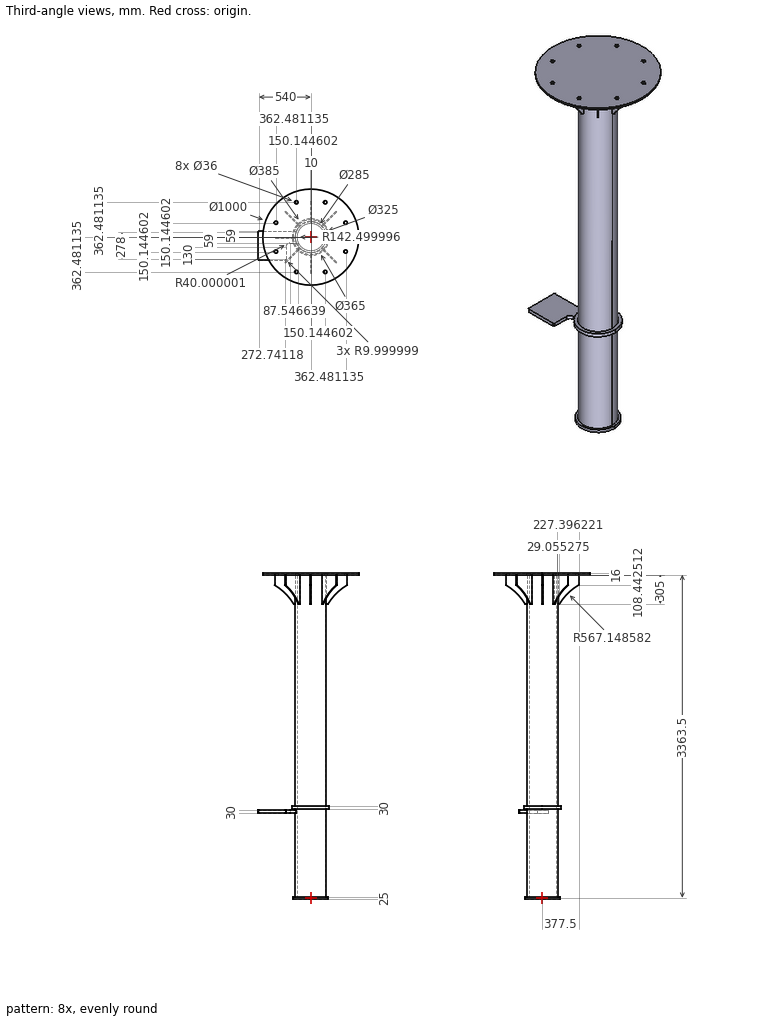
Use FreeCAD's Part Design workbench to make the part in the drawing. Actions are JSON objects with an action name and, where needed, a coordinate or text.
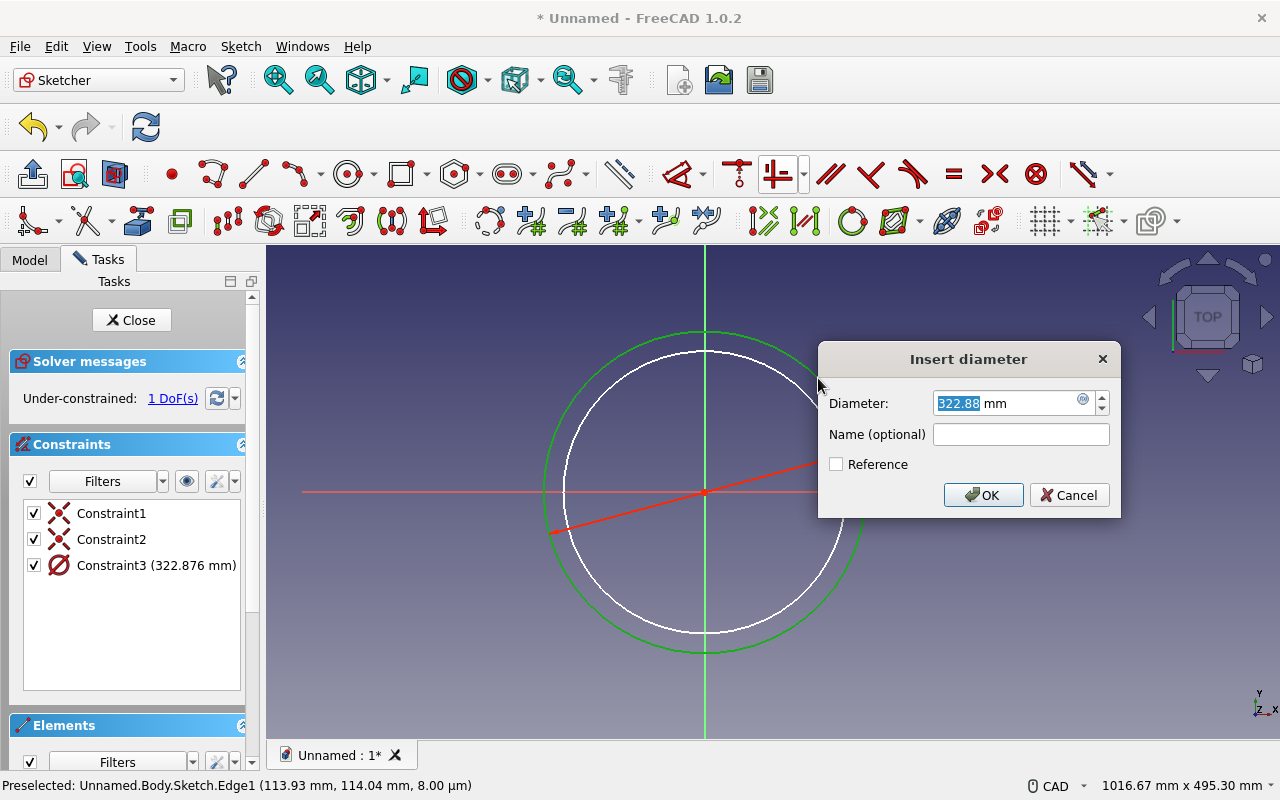
{"action": "type", "text": "325"}
{"action": "key", "text": "Return"}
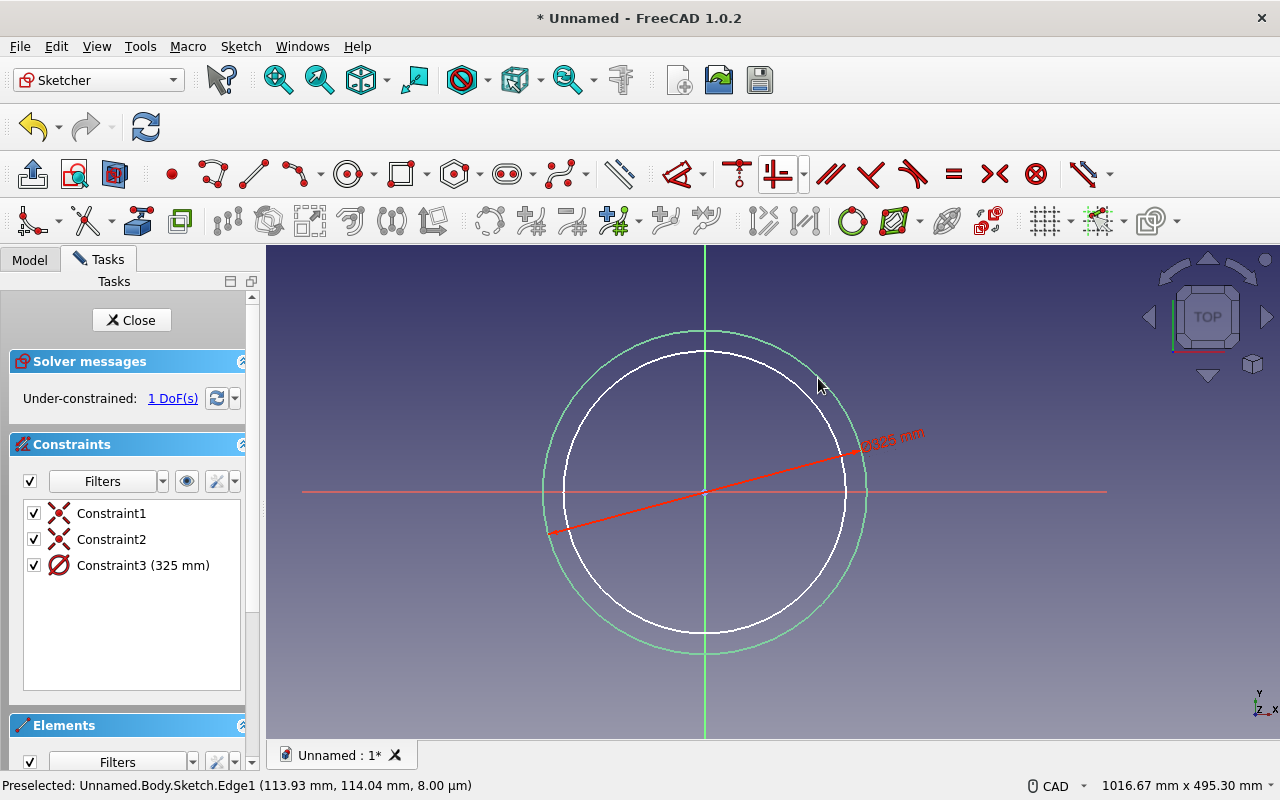
{"action": "left_click", "coordinate": [804, 392]}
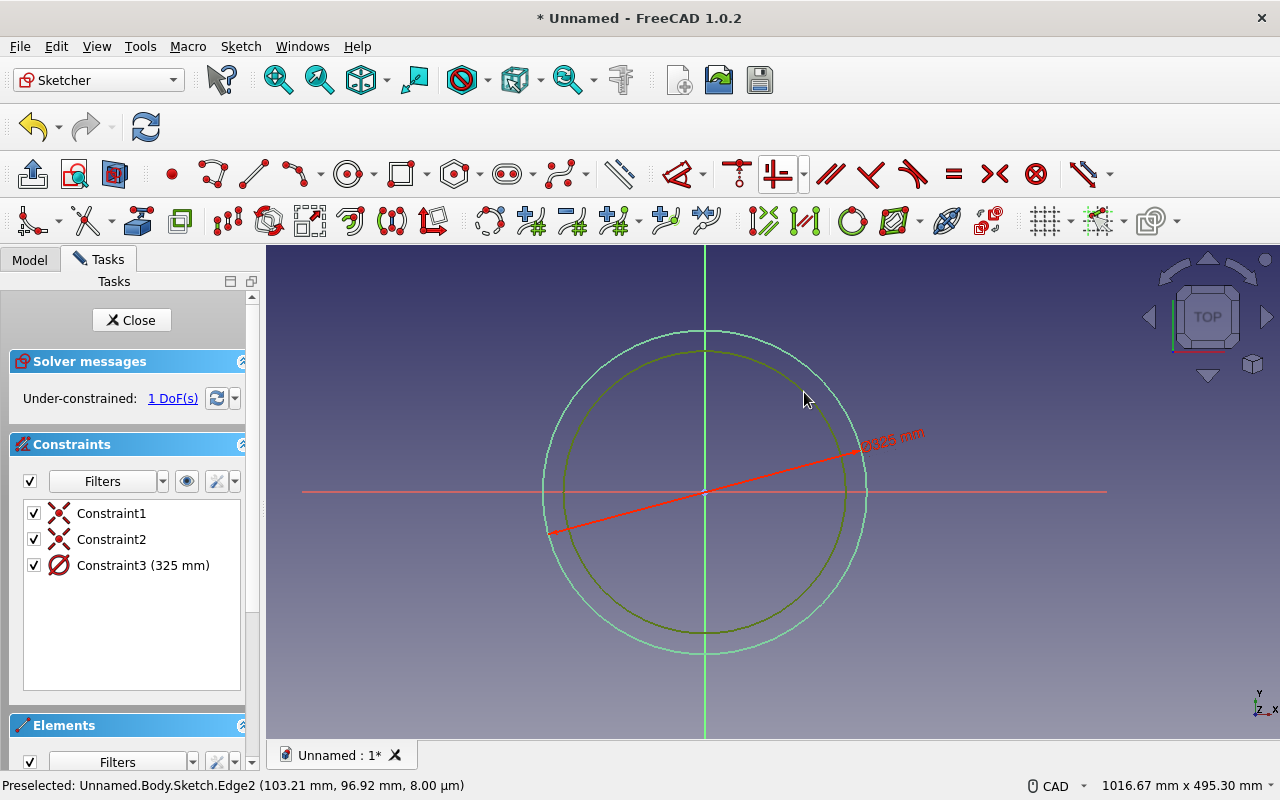
{"action": "key", "text": "k o"}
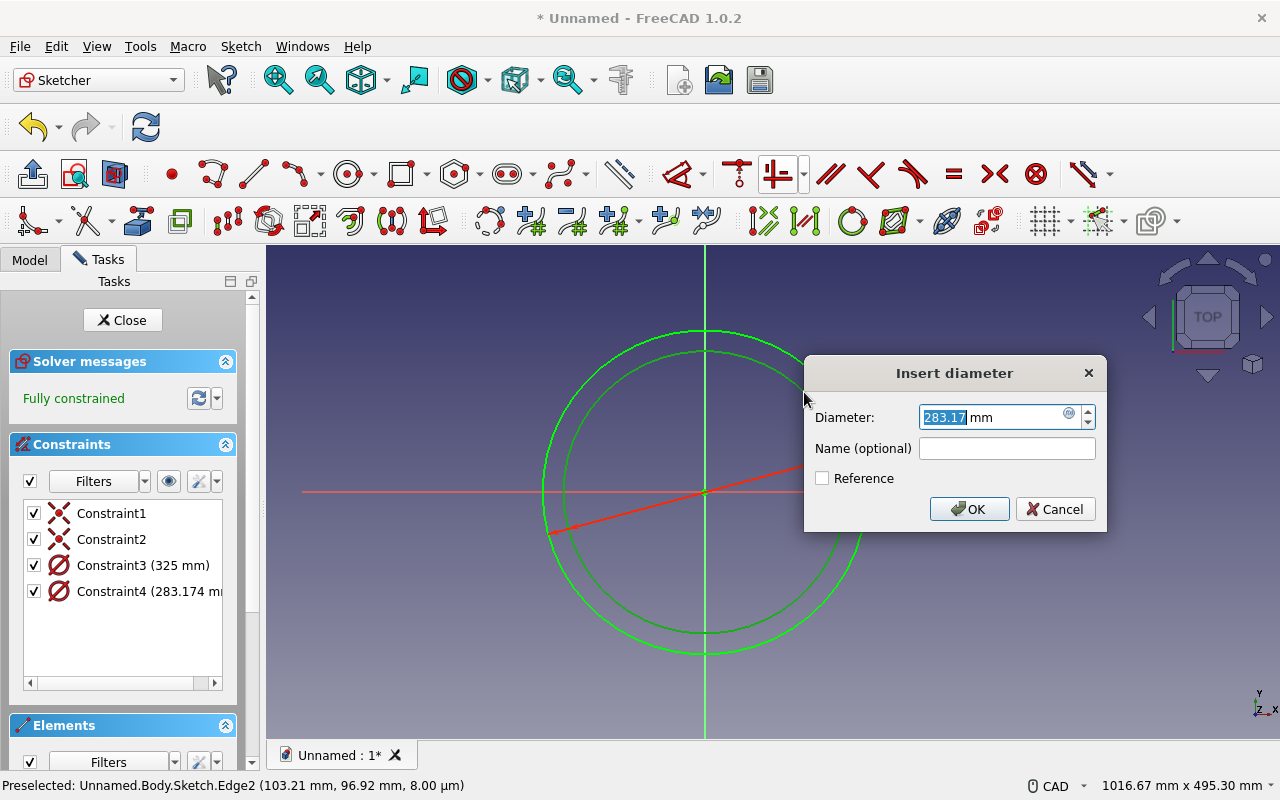
{"action": "type", "text": "285"}
{"action": "key", "text": "Return"}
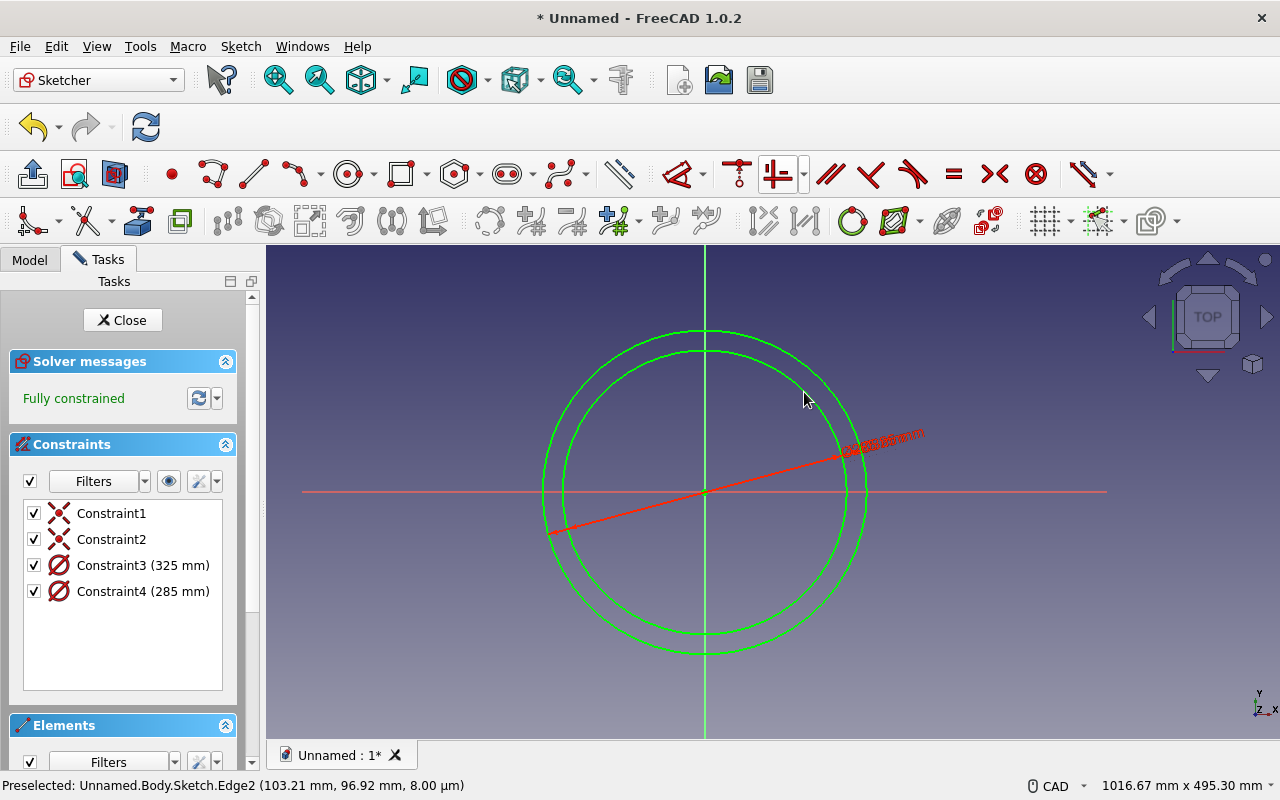
{"action": "left_click", "coordinate": [123, 320]}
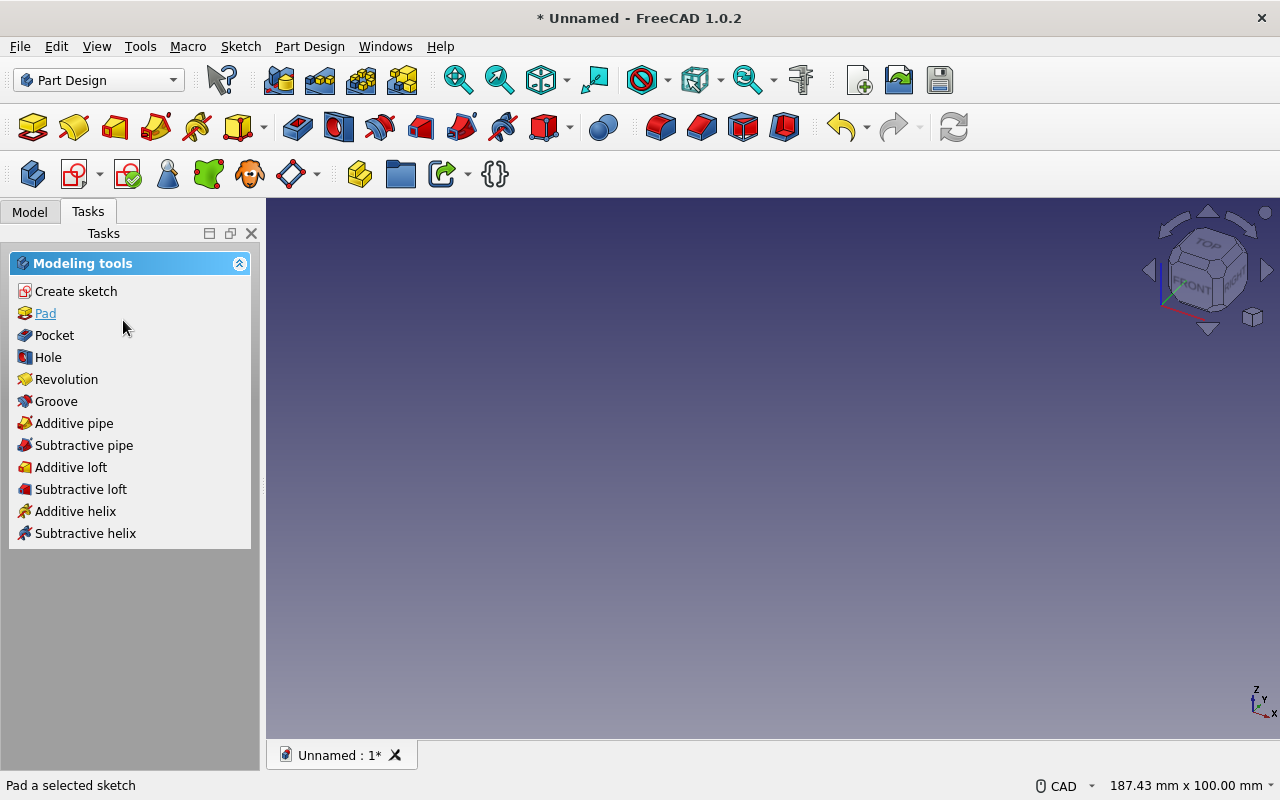
{"action": "left_click", "coordinate": [33, 128]}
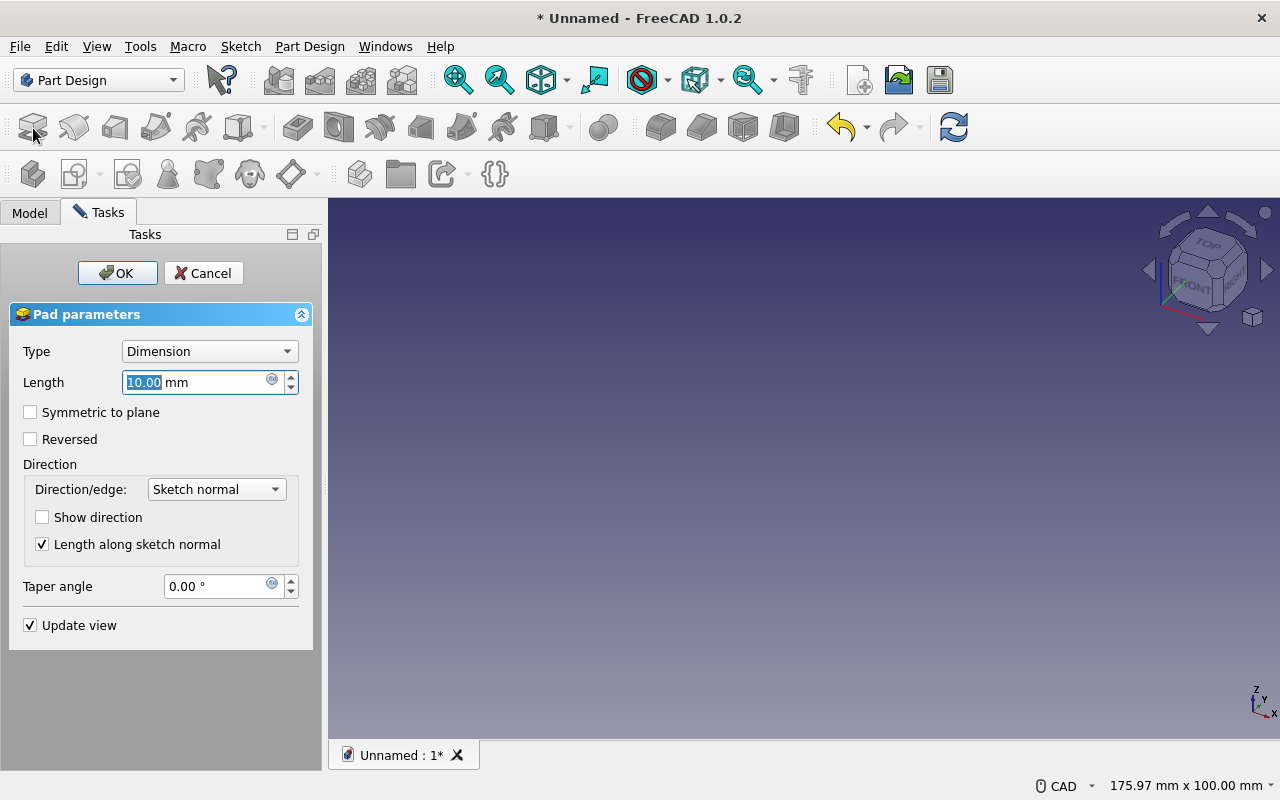
{"action": "type", "text": "3363.5"}
{"action": "key", "text": "Tab"}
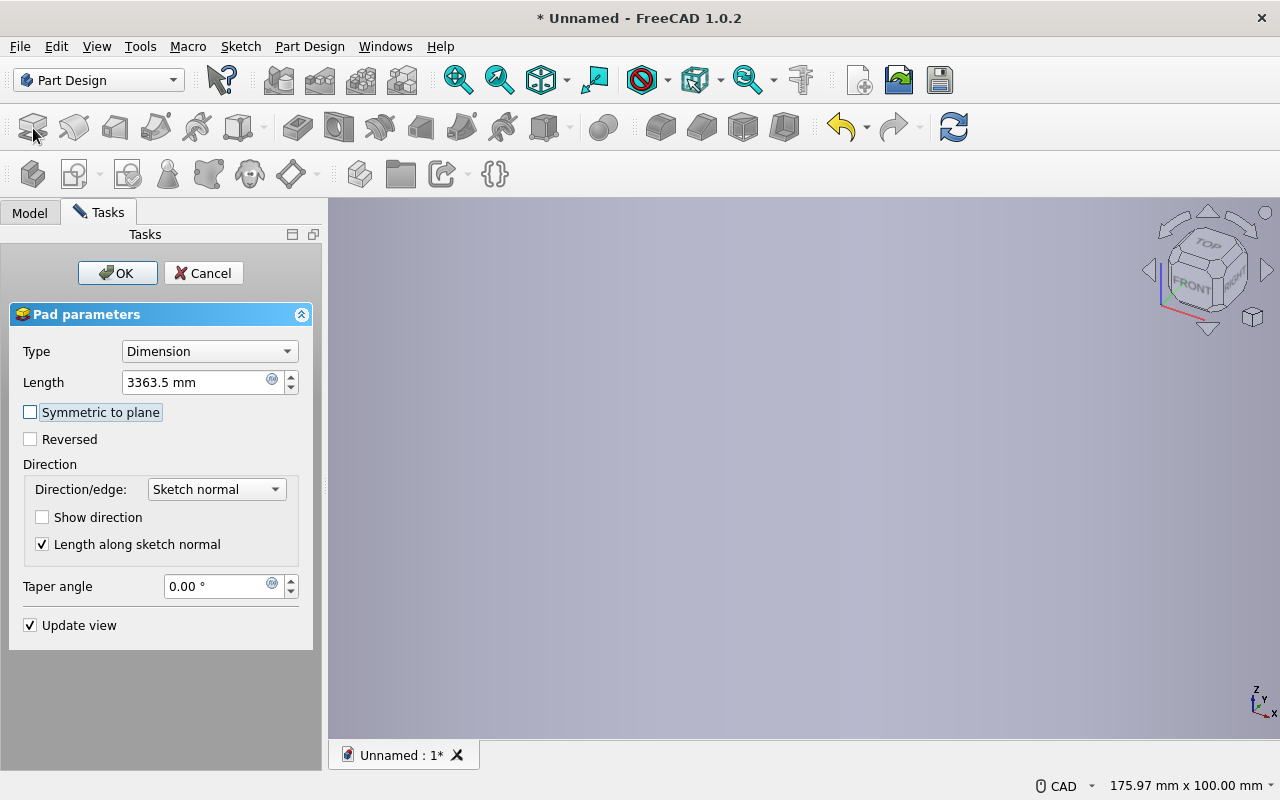
{"action": "left_click", "coordinate": [118, 273]}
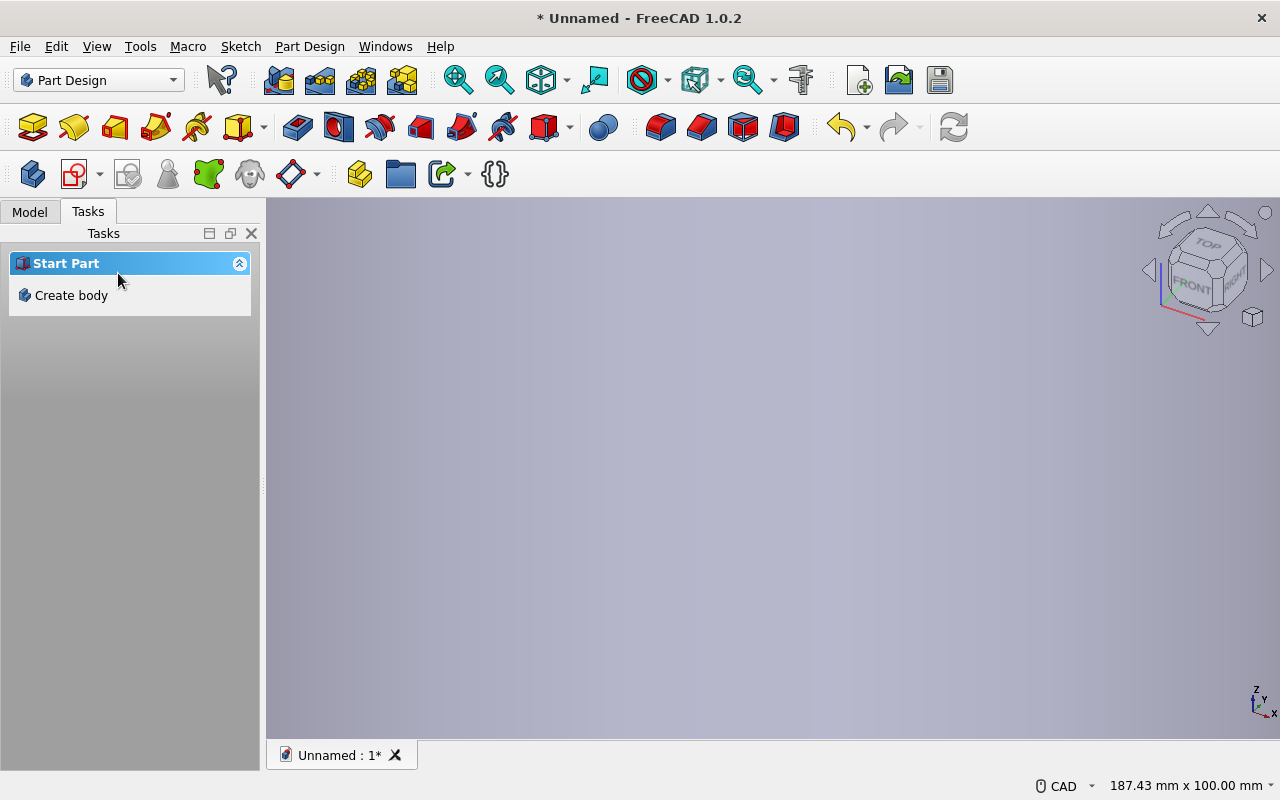
{"action": "key", "text": "v f"}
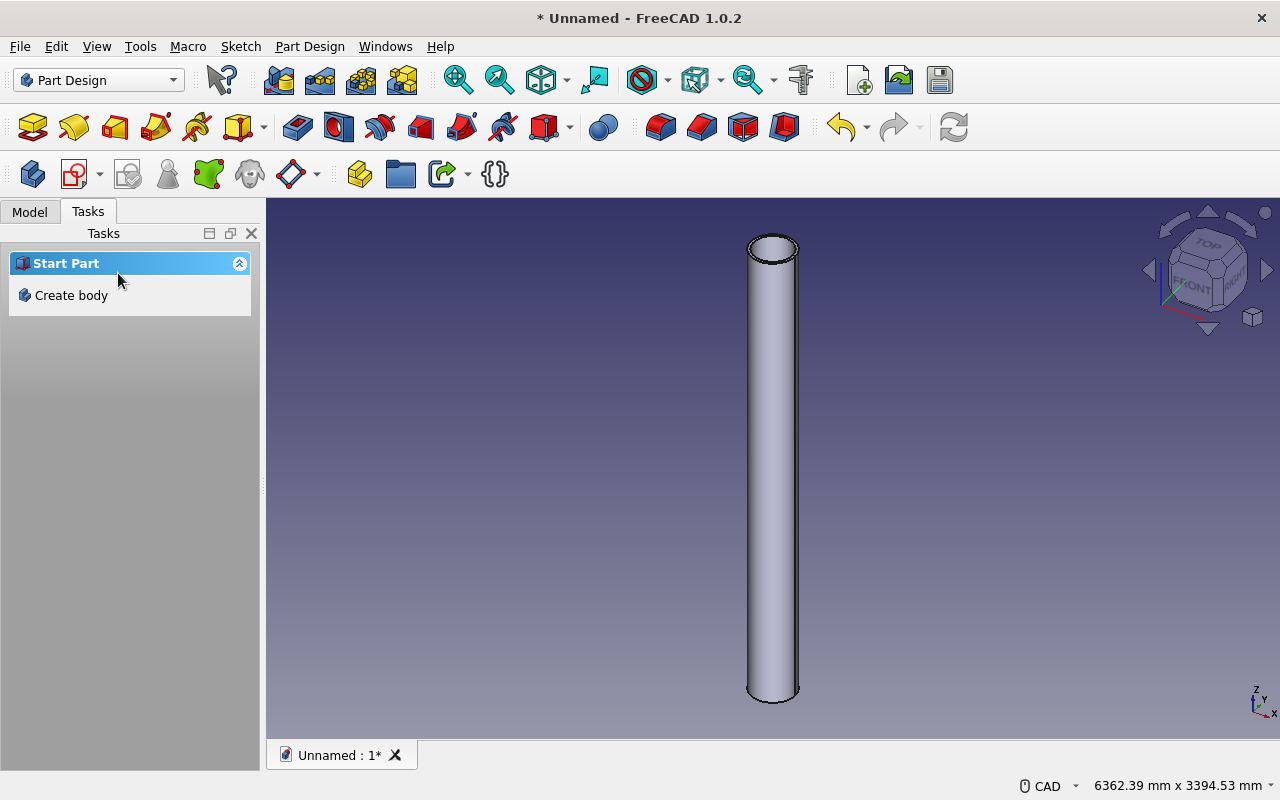
{"action": "left_click", "coordinate": [30, 212]}